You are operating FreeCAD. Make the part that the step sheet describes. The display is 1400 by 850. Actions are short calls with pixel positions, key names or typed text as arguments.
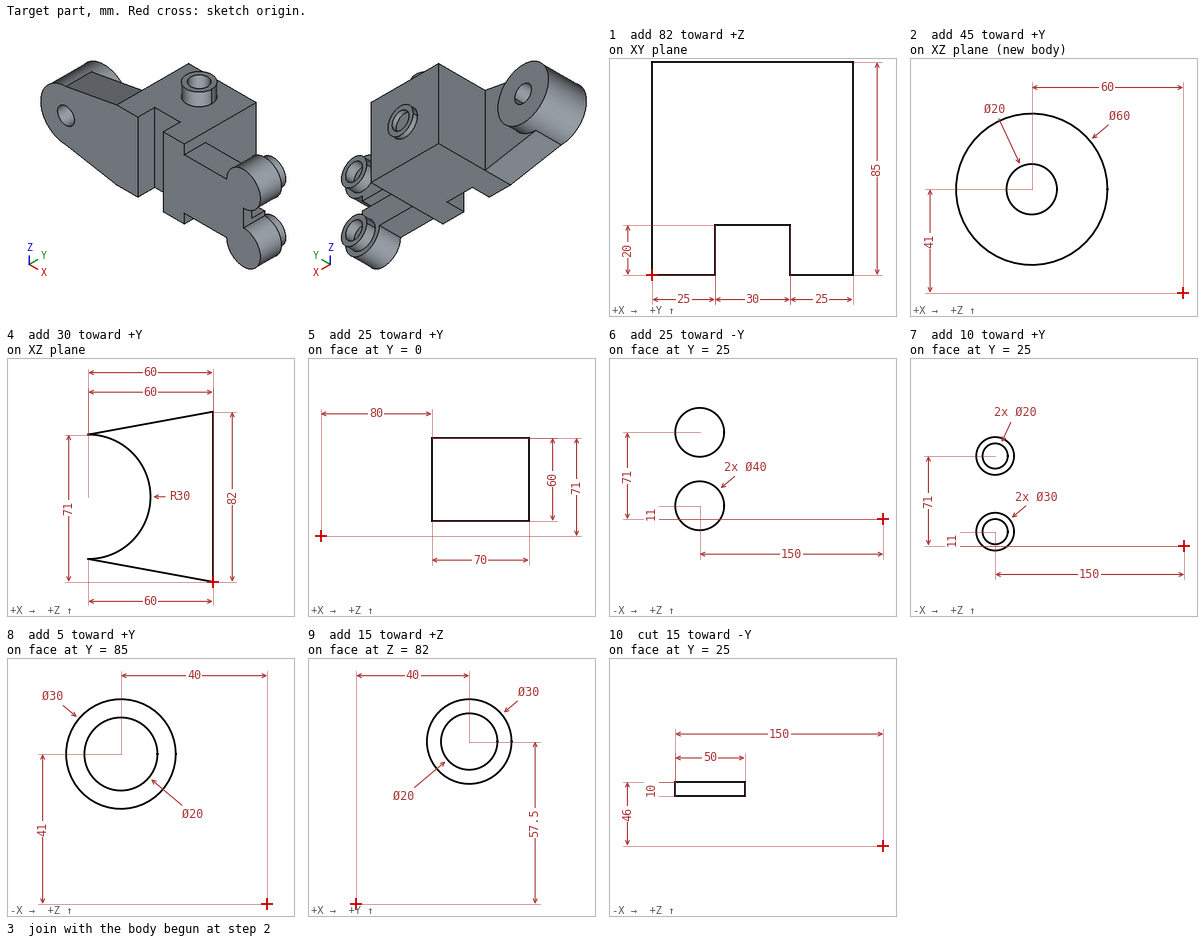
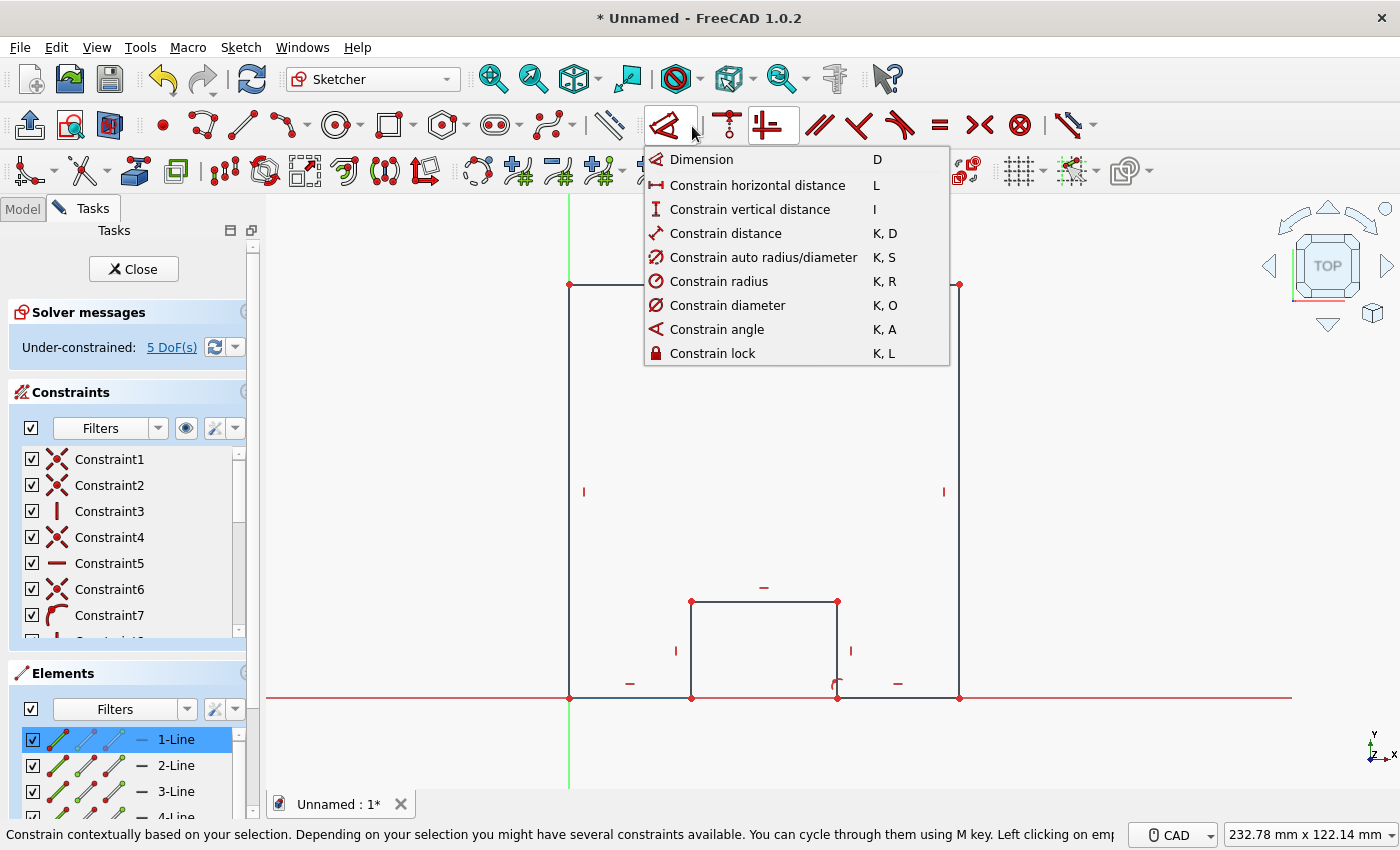
click(797, 185)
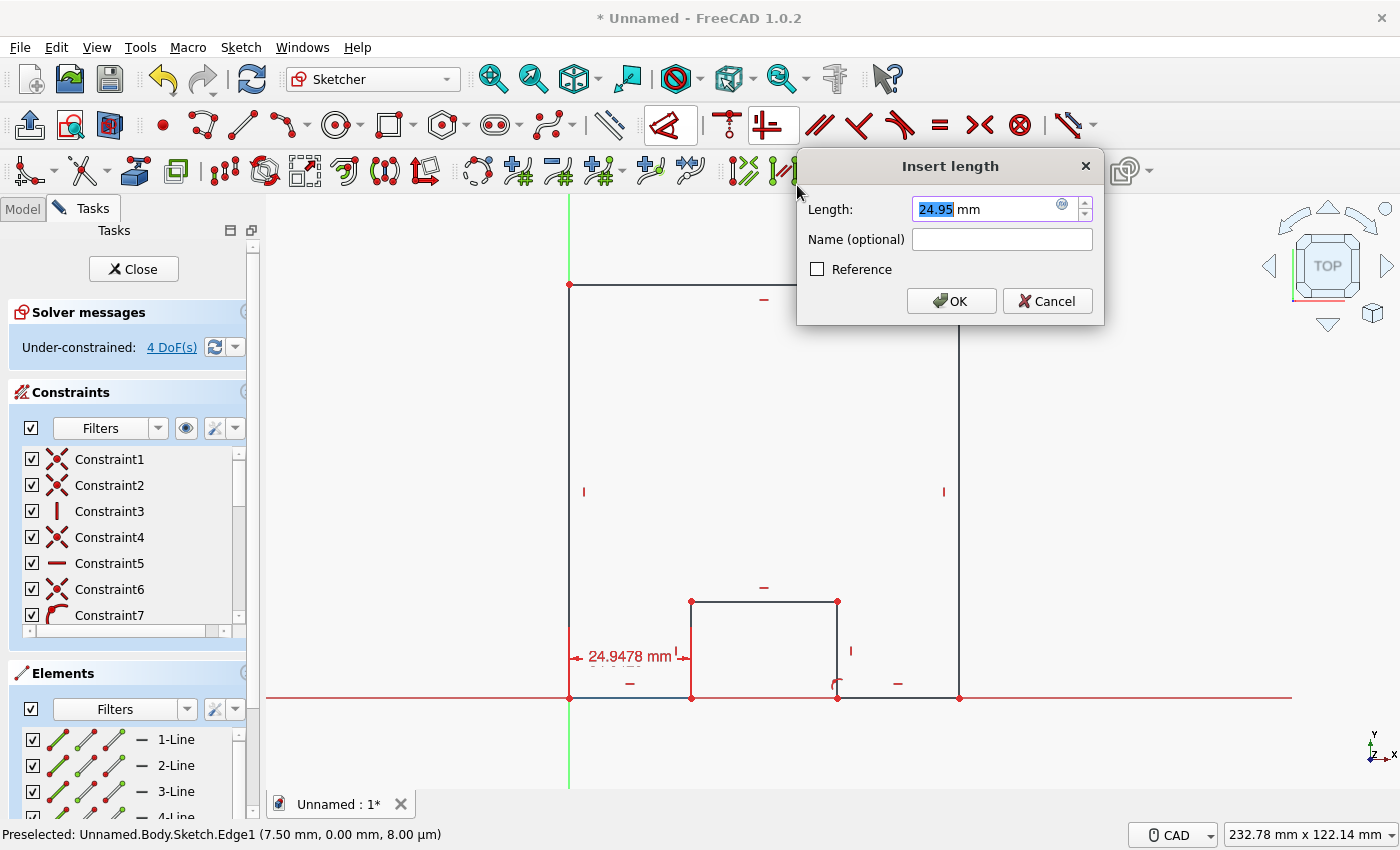
text(25)
key(Return)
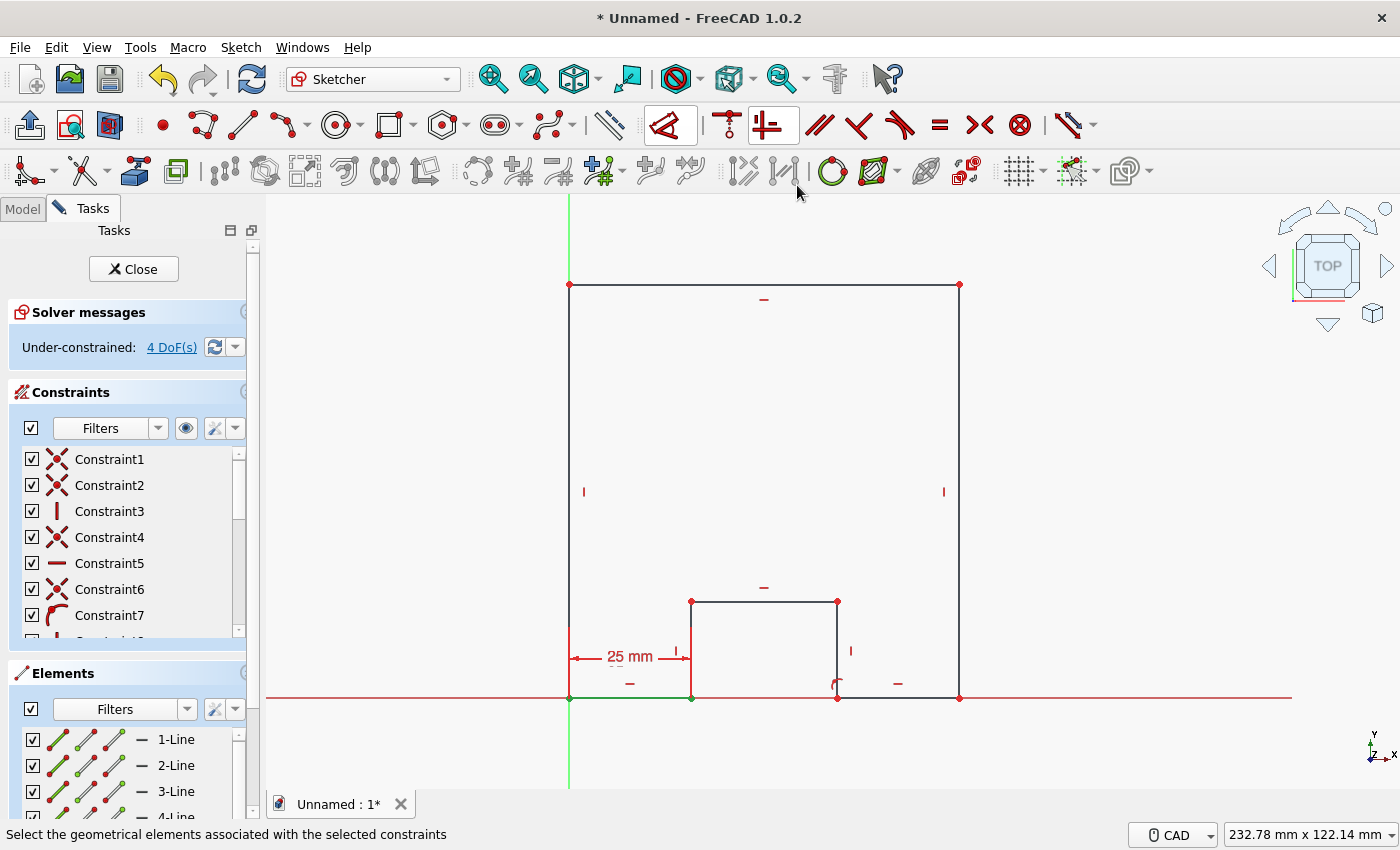
click(691, 669)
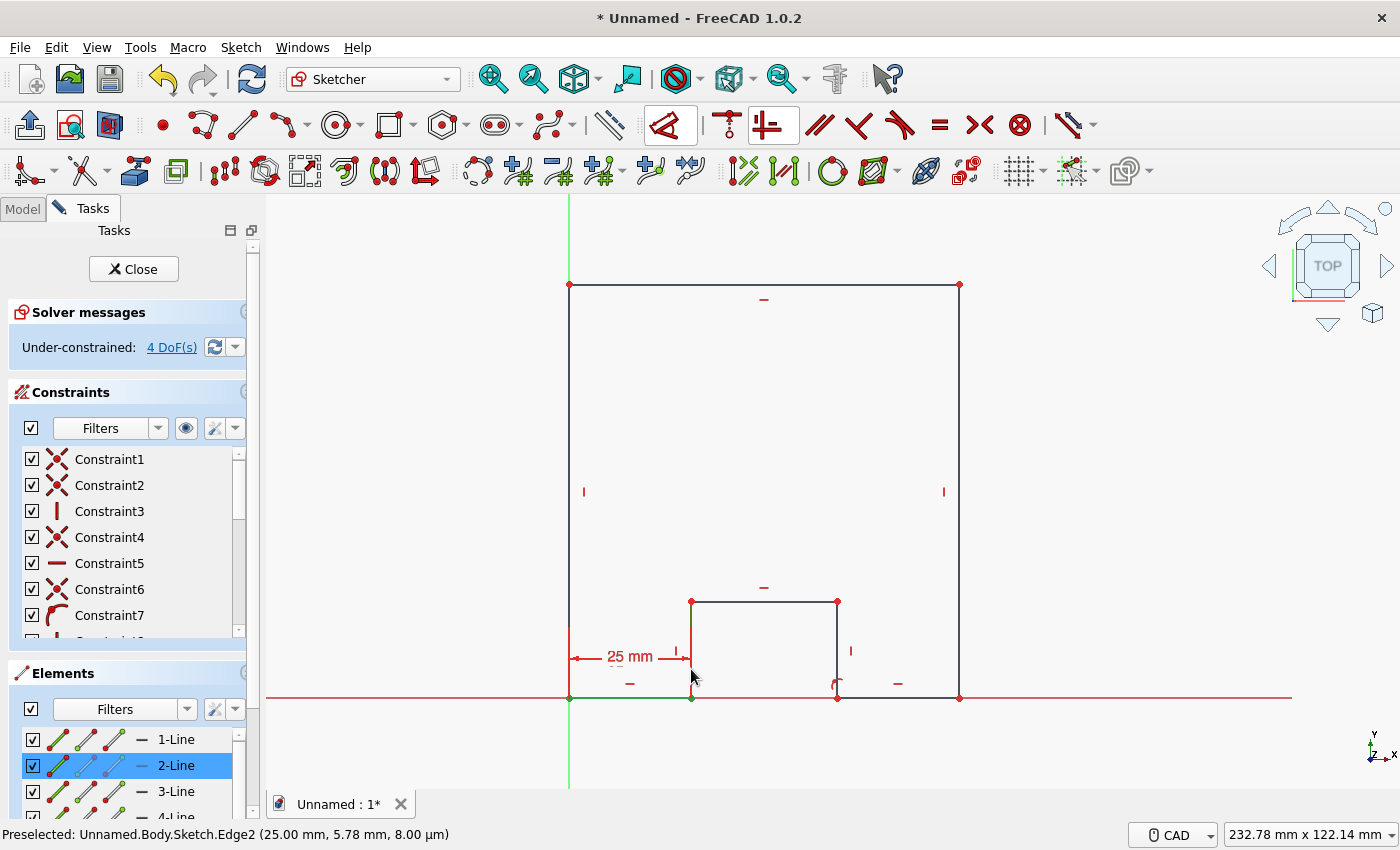
key(i)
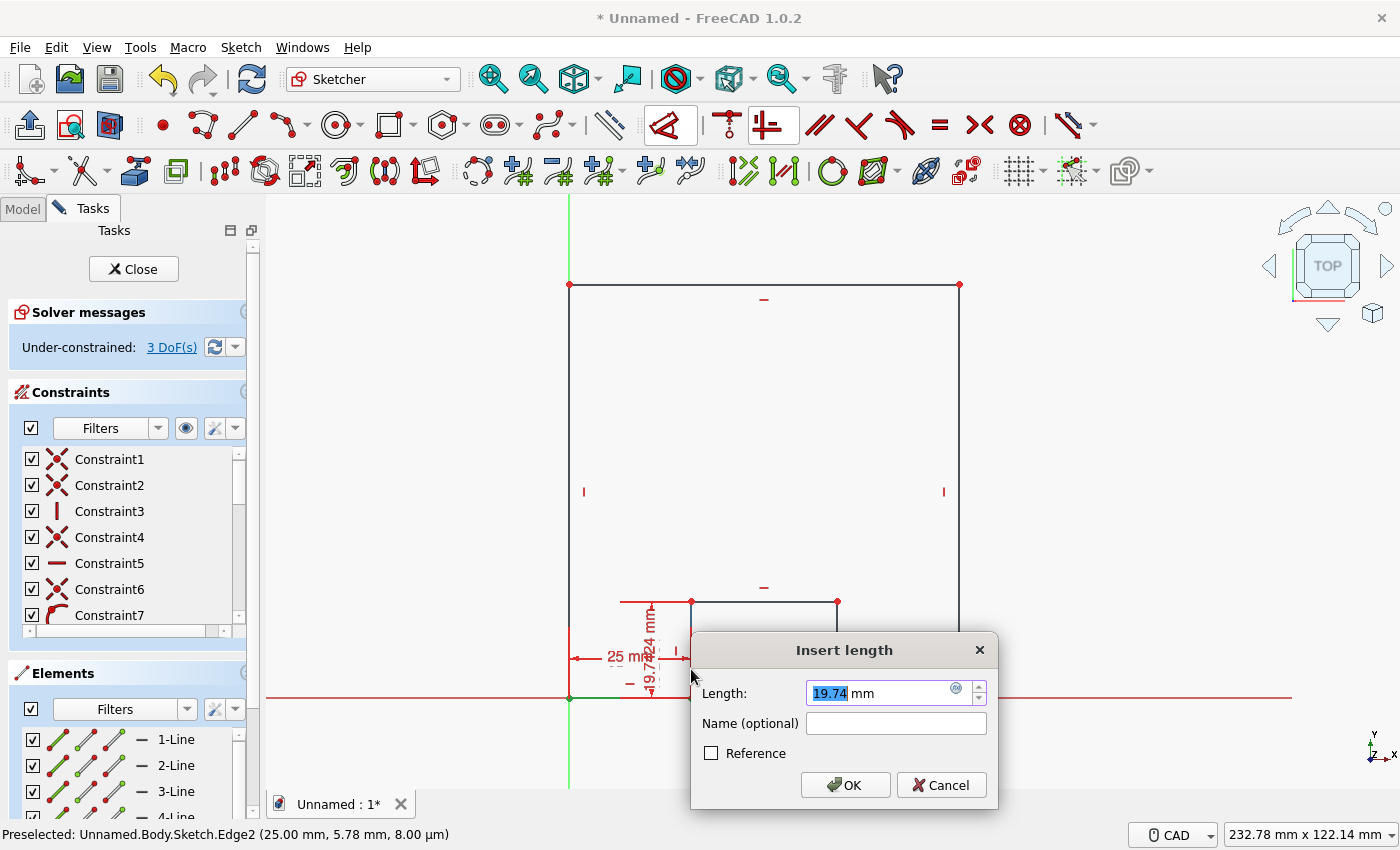
text(20)
key(Return)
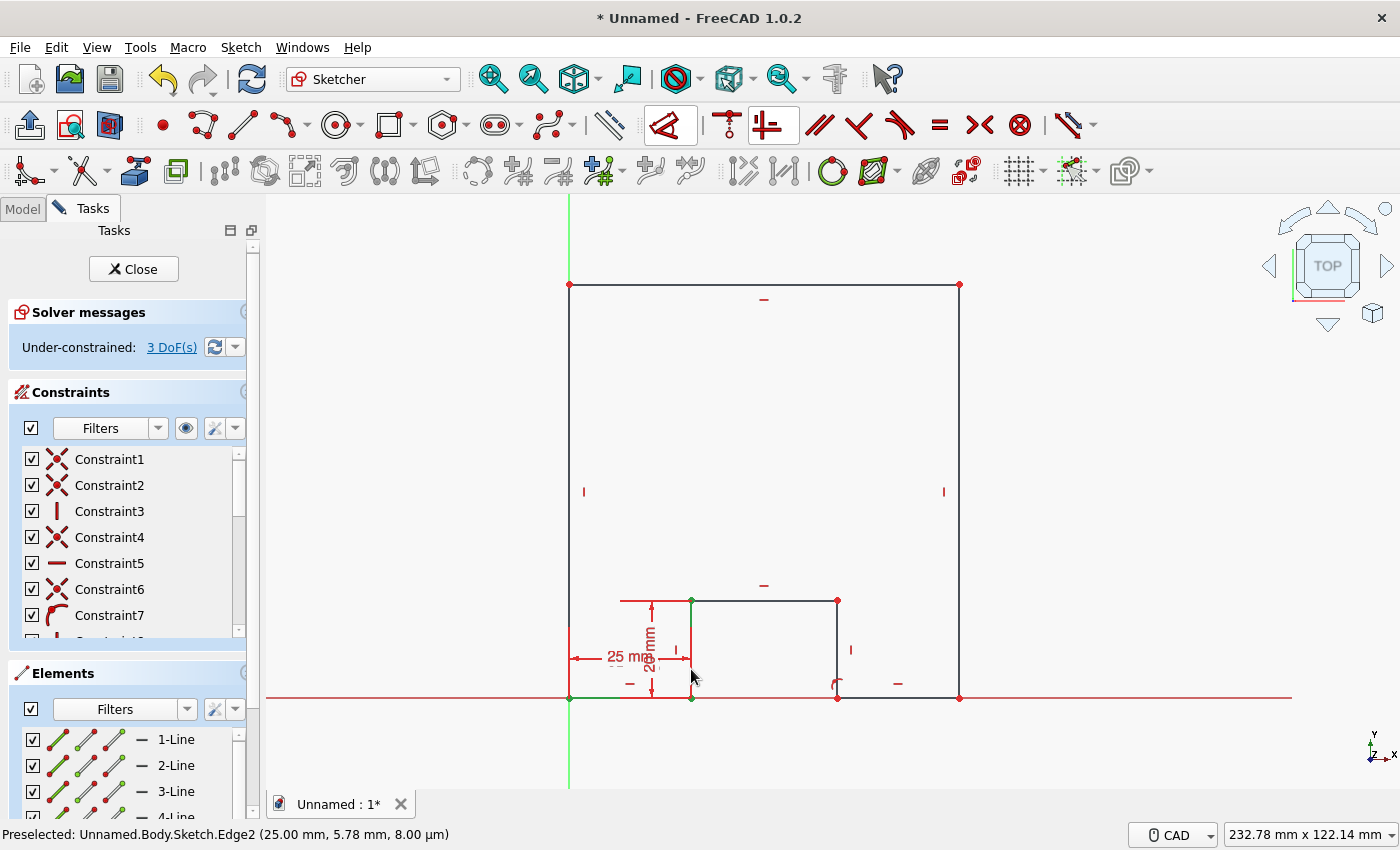
click(735, 601)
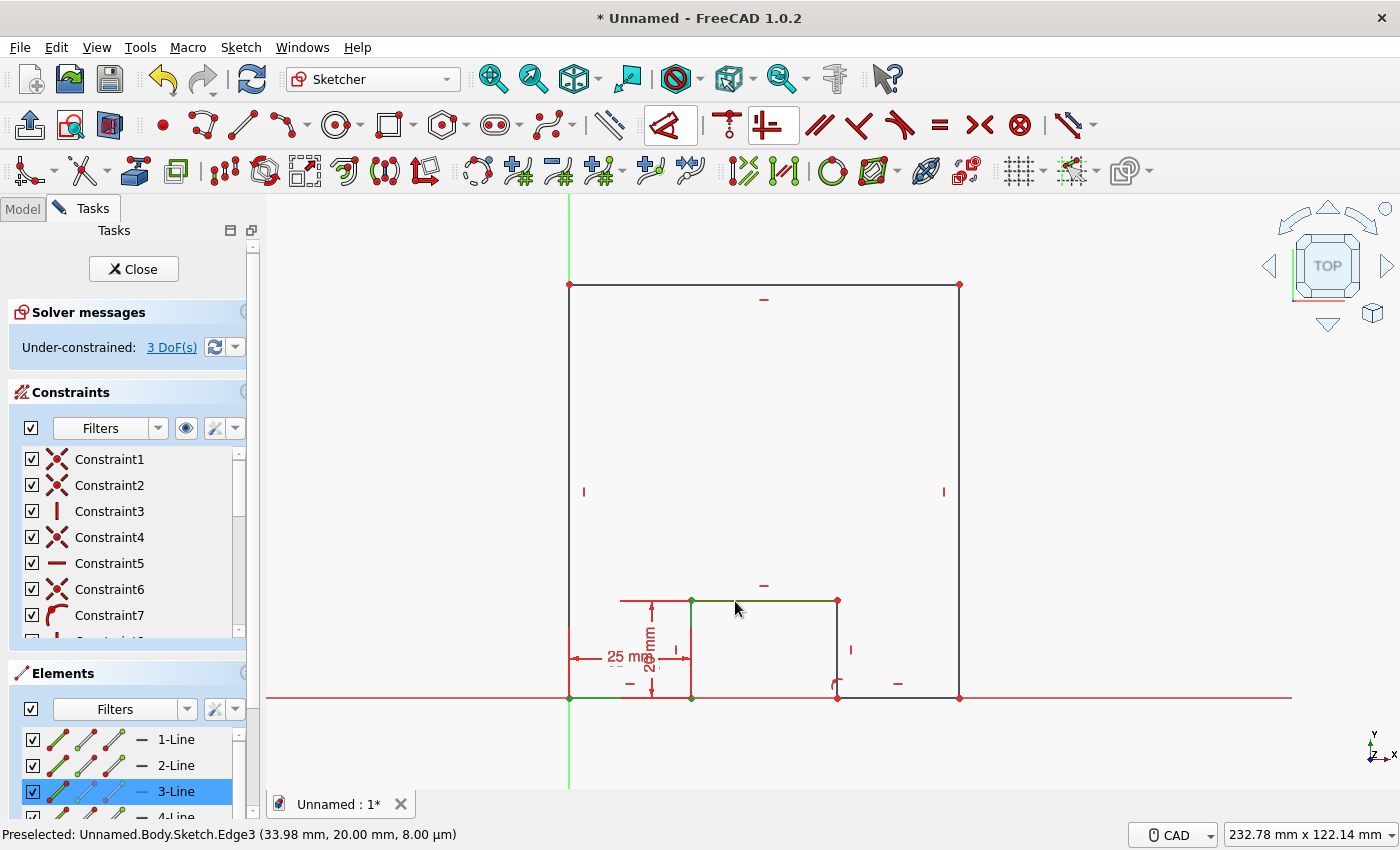
key(l)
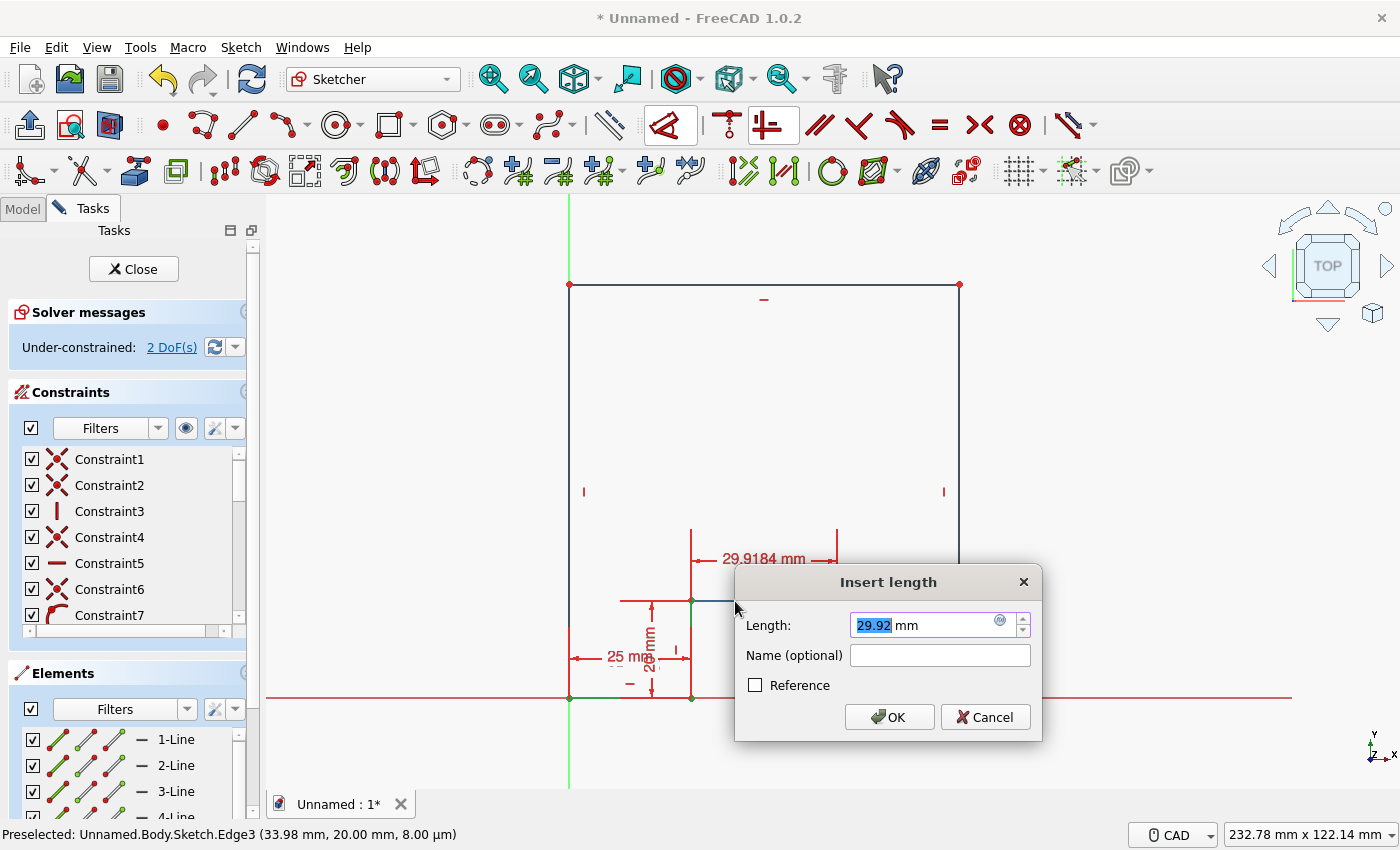
text(30)
key(Return)